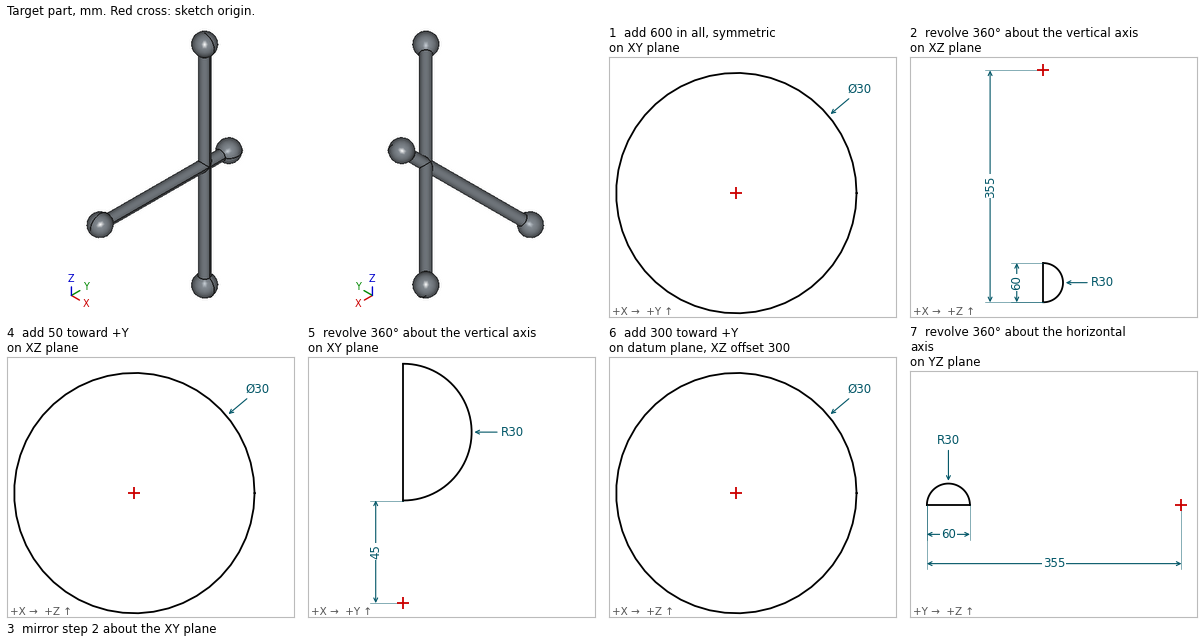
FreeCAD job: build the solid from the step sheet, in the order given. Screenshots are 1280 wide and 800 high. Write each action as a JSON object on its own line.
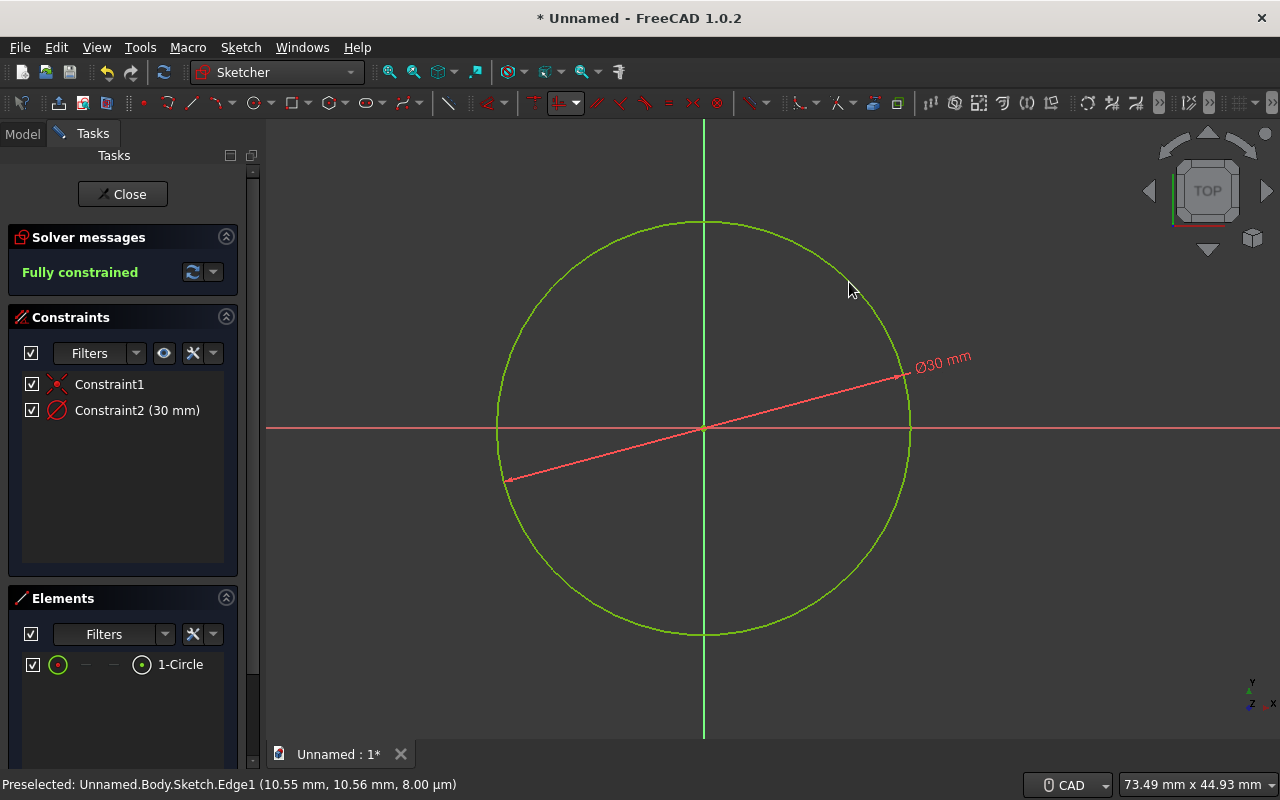
{"action": "left_click", "coordinate": [123, 194]}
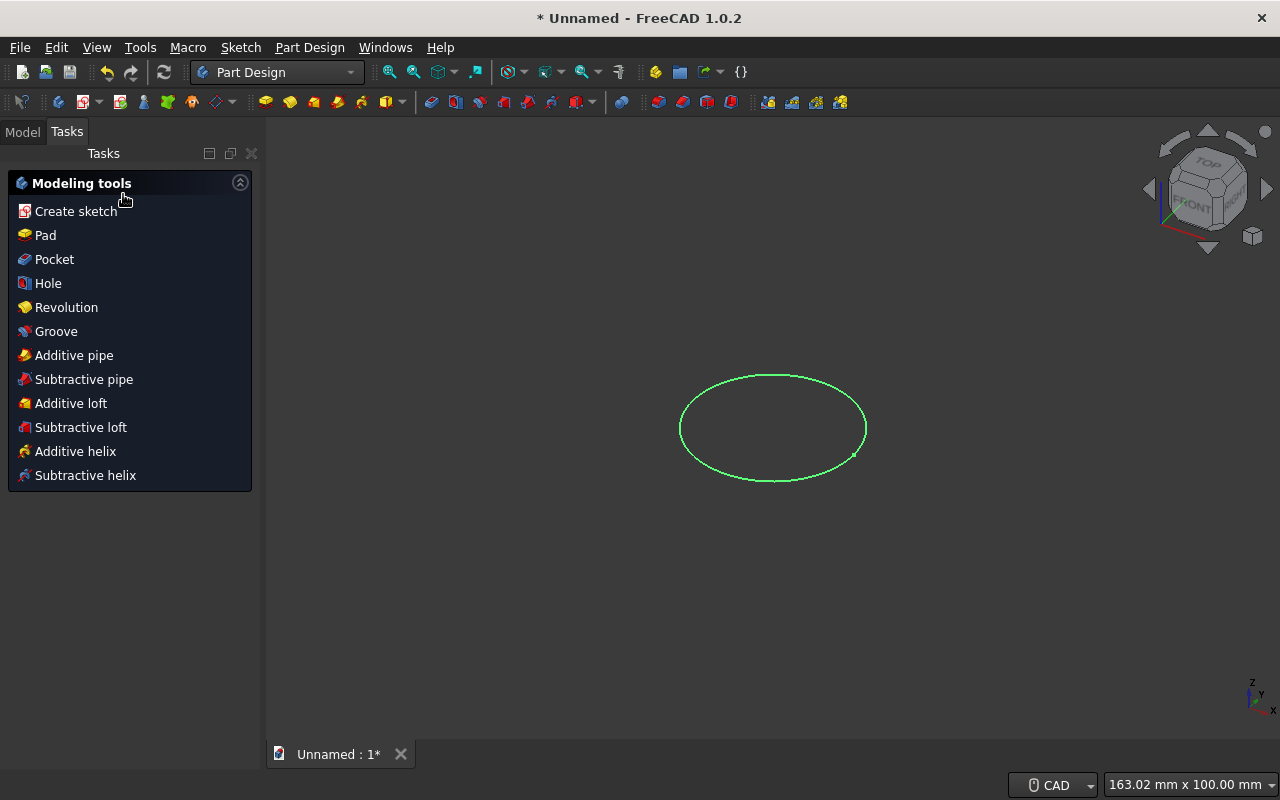
{"action": "left_click", "coordinate": [266, 102]}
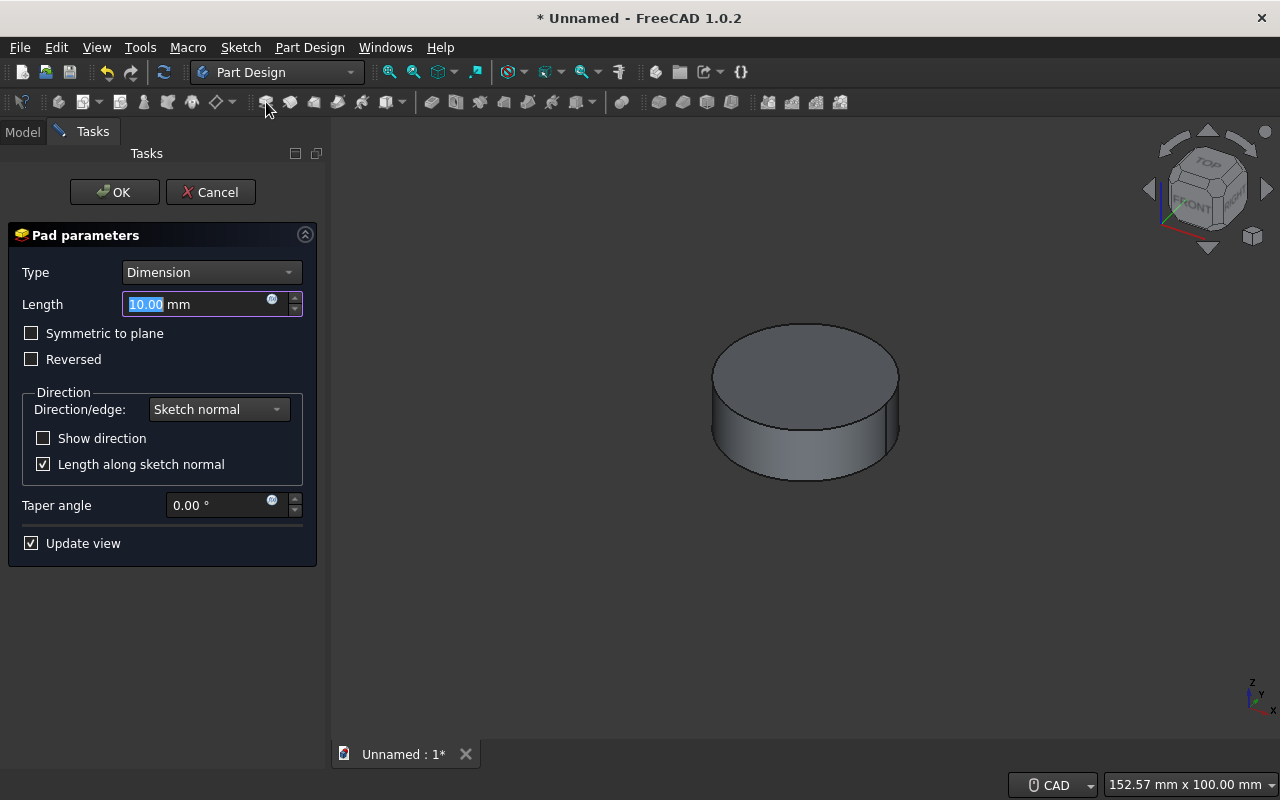
{"action": "type", "text": "600"}
{"action": "key", "text": "Tab"}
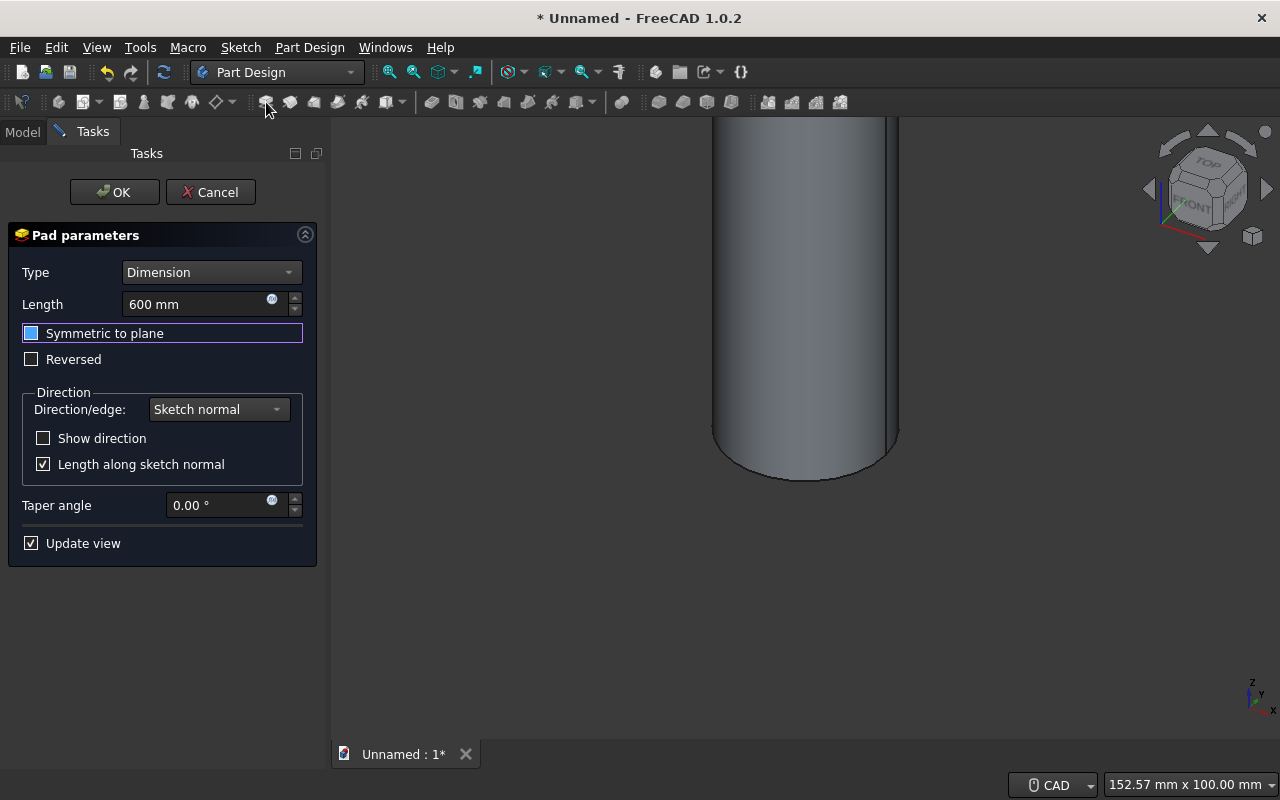
{"action": "left_click", "coordinate": [30, 333]}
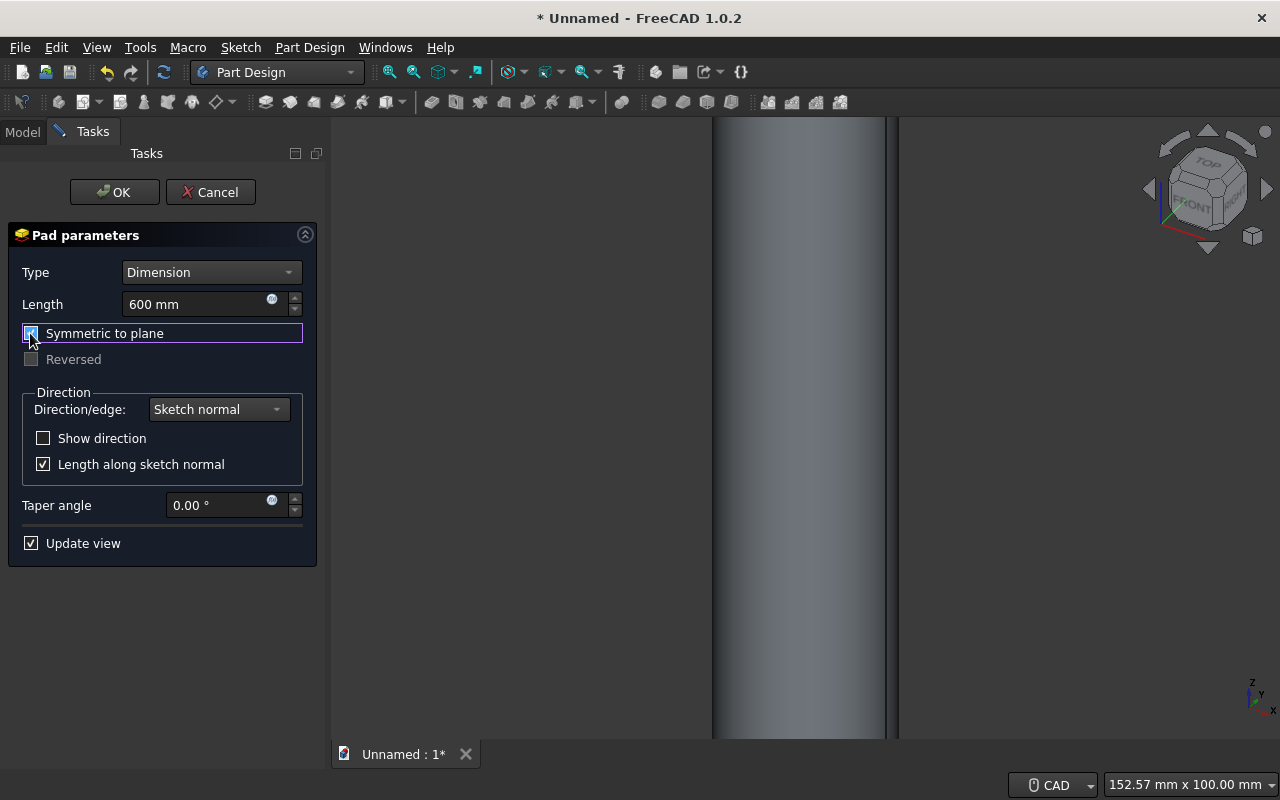
{"action": "left_click", "coordinate": [115, 192]}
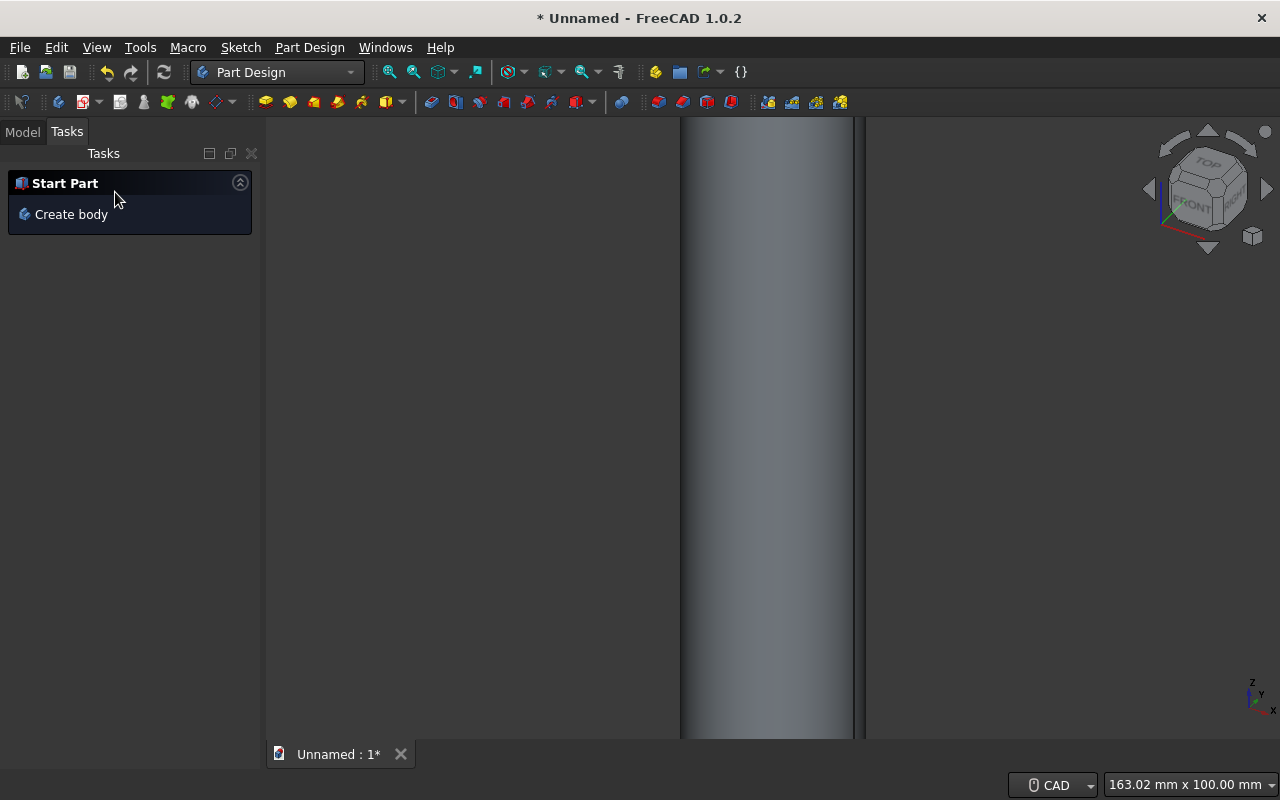
{"action": "left_click", "coordinate": [390, 72]}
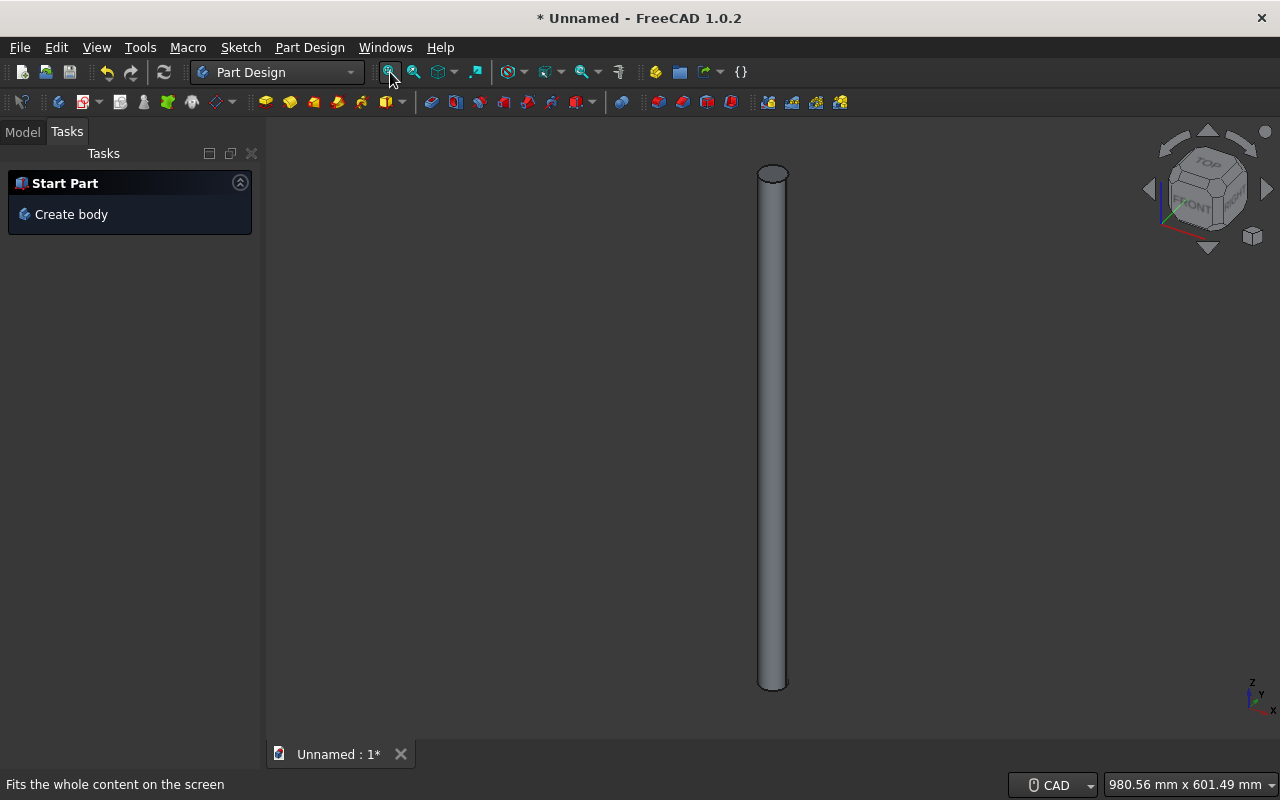
{"action": "left_click", "coordinate": [84, 102]}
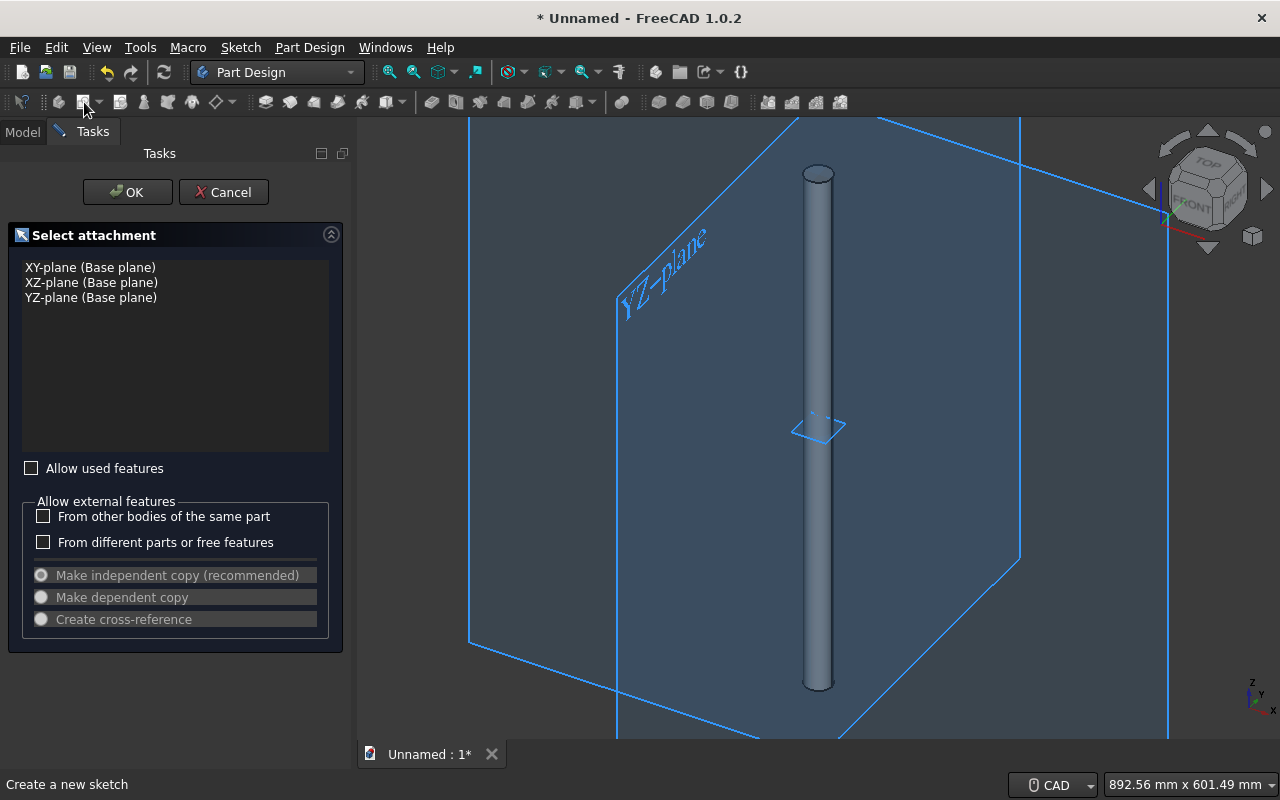
{"action": "left_click", "coordinate": [82, 282]}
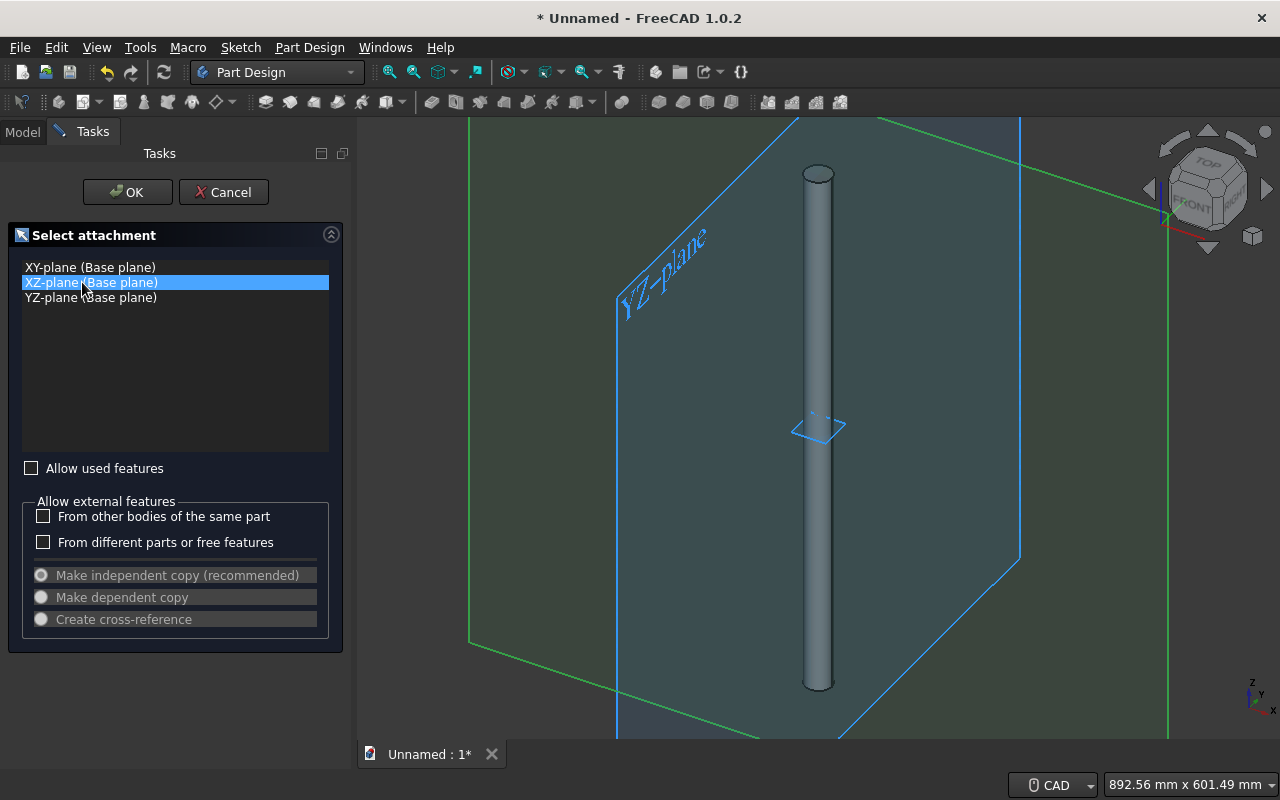
{"action": "left_click", "coordinate": [128, 192]}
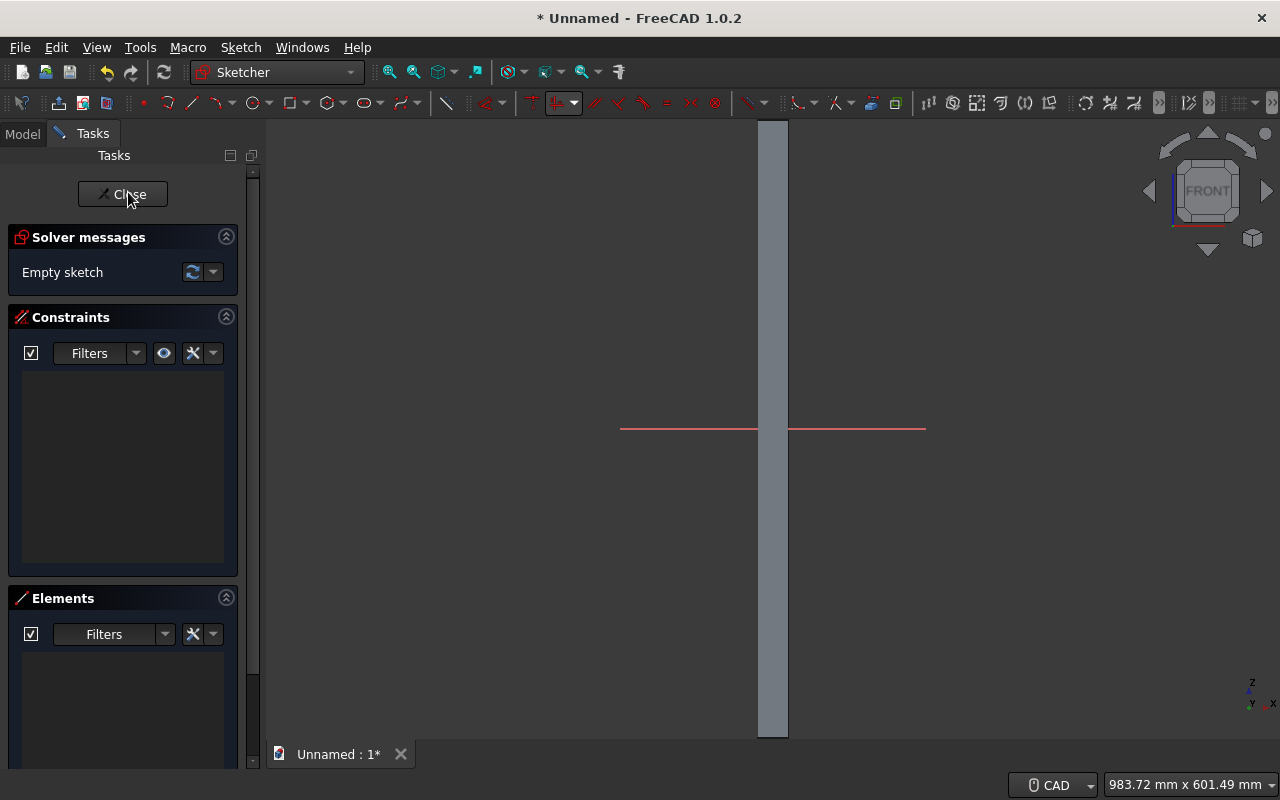
{"action": "key", "text": "q s"}